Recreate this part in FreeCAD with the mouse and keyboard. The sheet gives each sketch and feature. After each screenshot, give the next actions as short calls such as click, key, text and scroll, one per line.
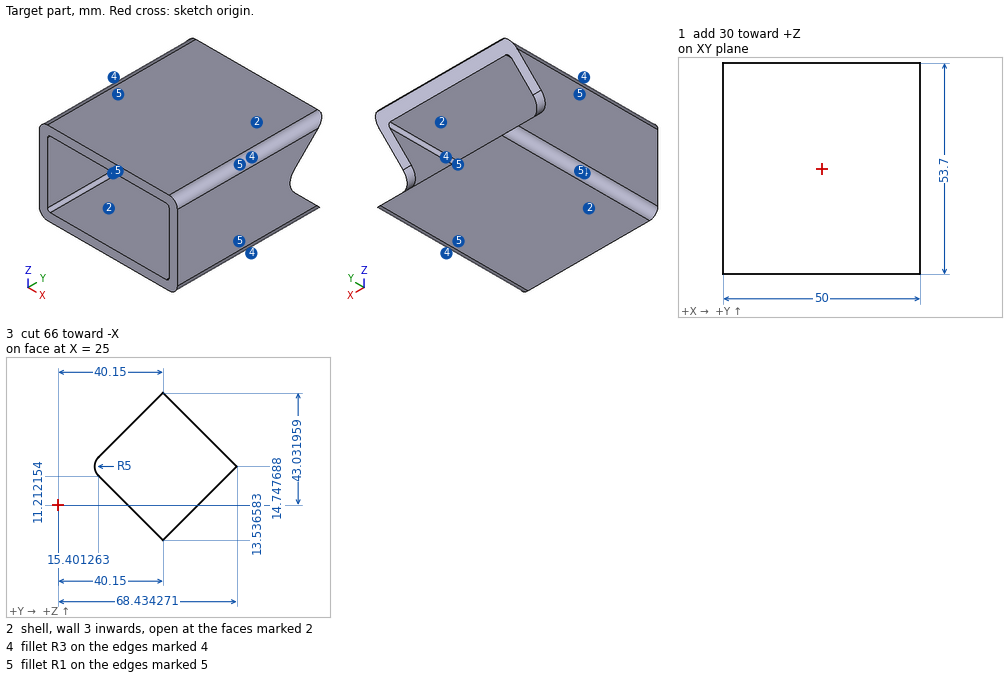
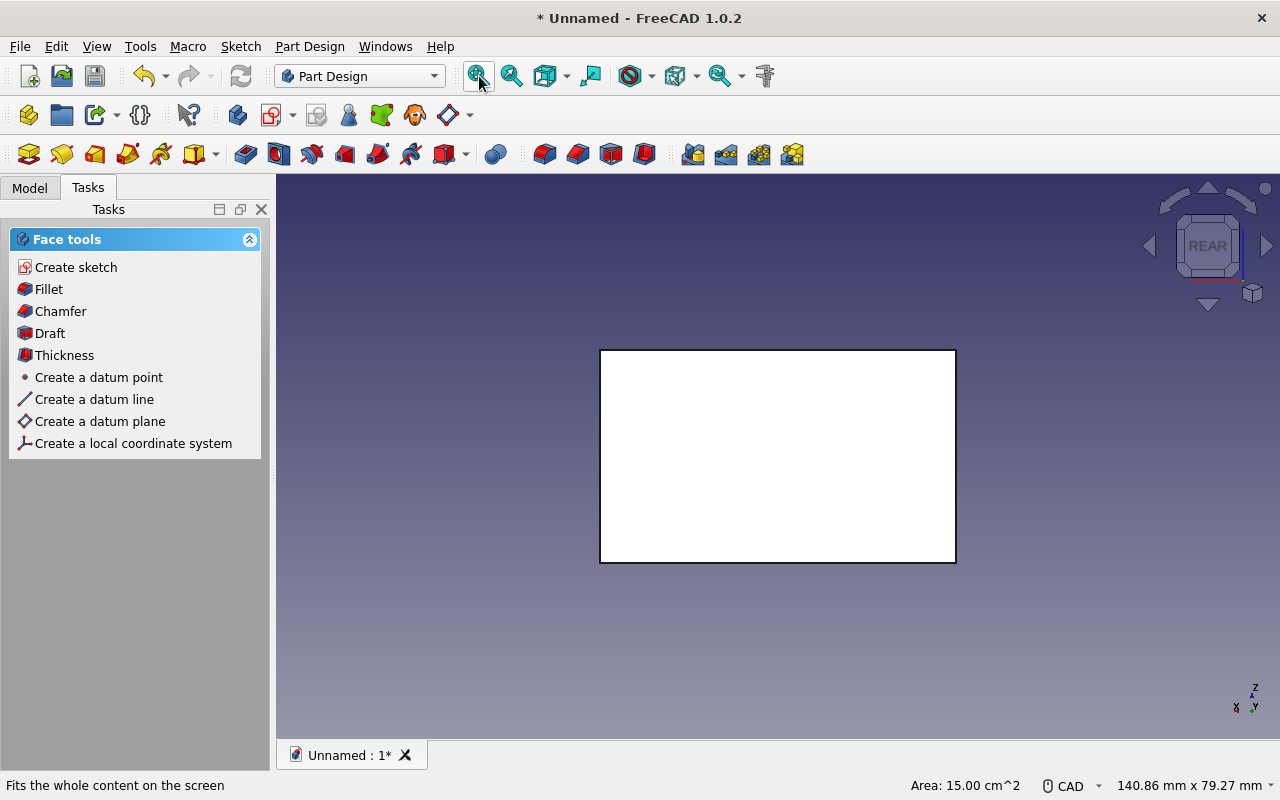
click(479, 76)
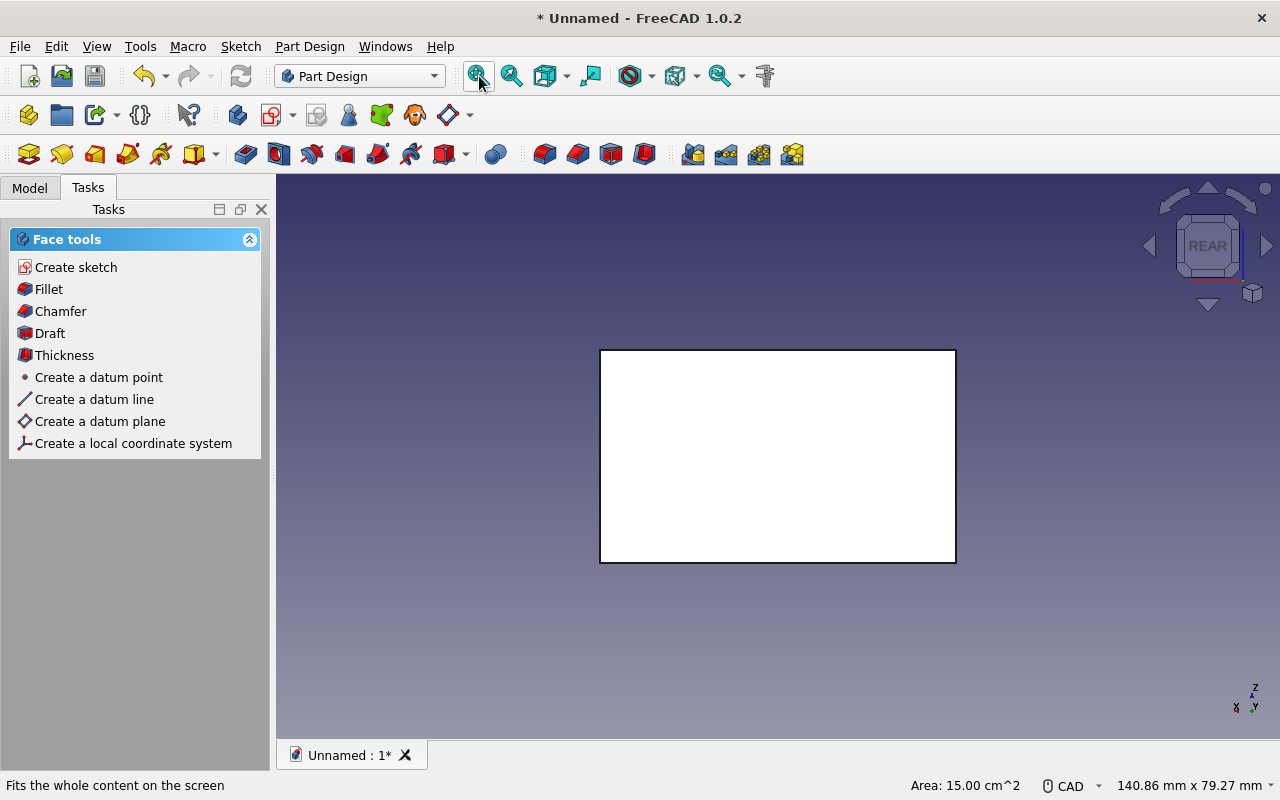
click(727, 456, ctrl)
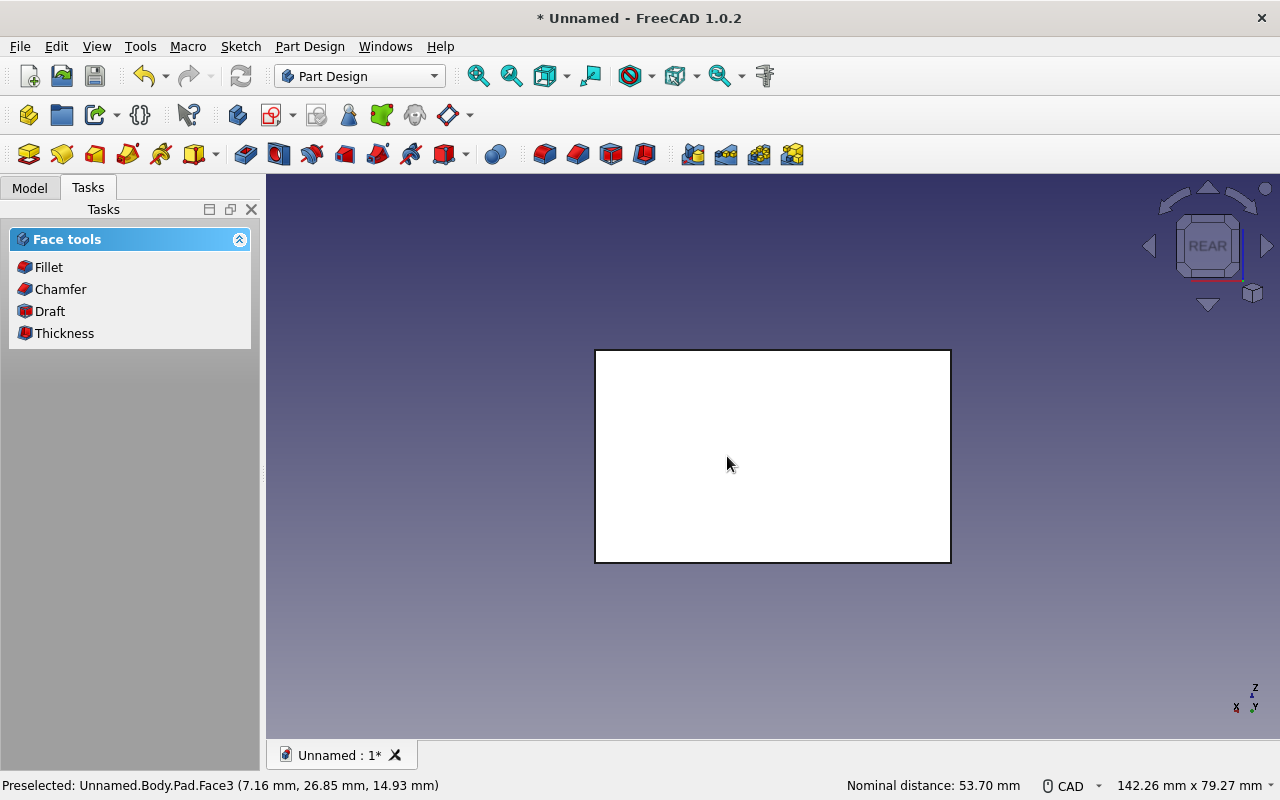
click(644, 154)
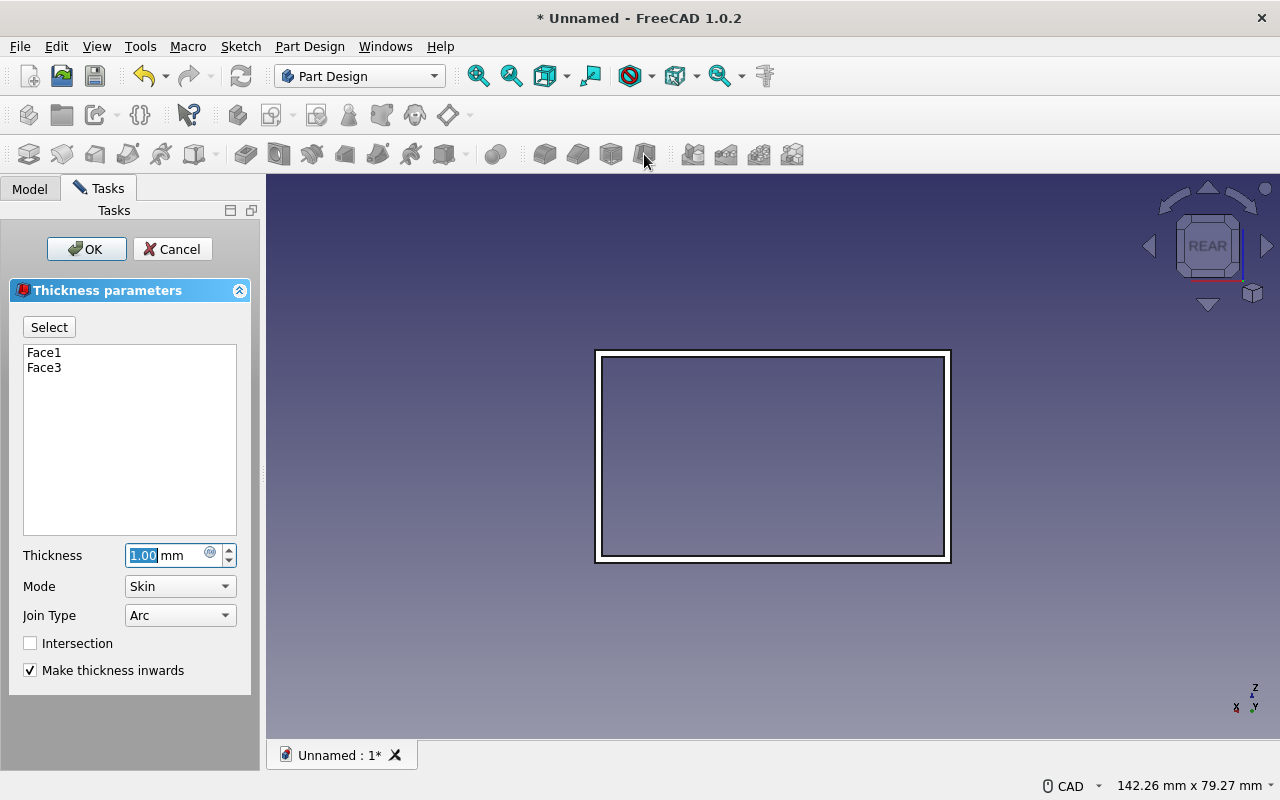
text(3)
key(Tab)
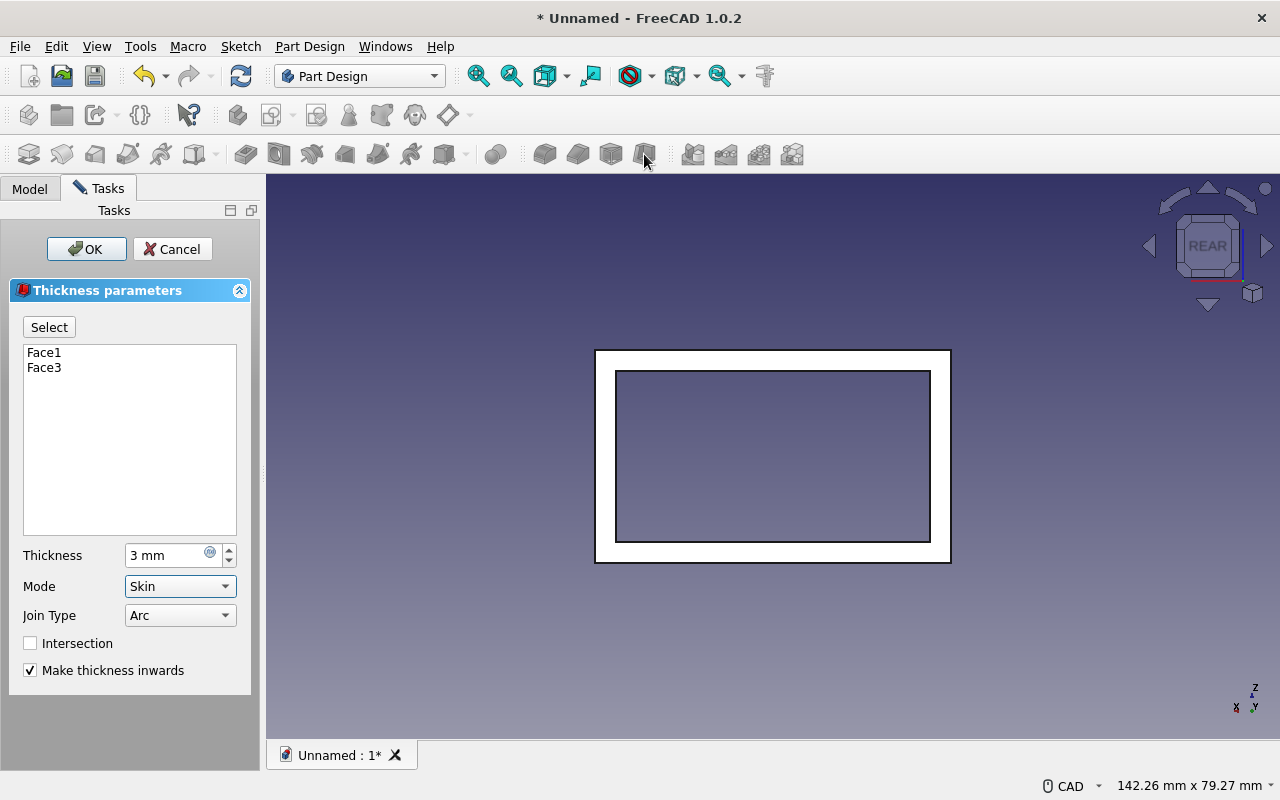
click(181, 616)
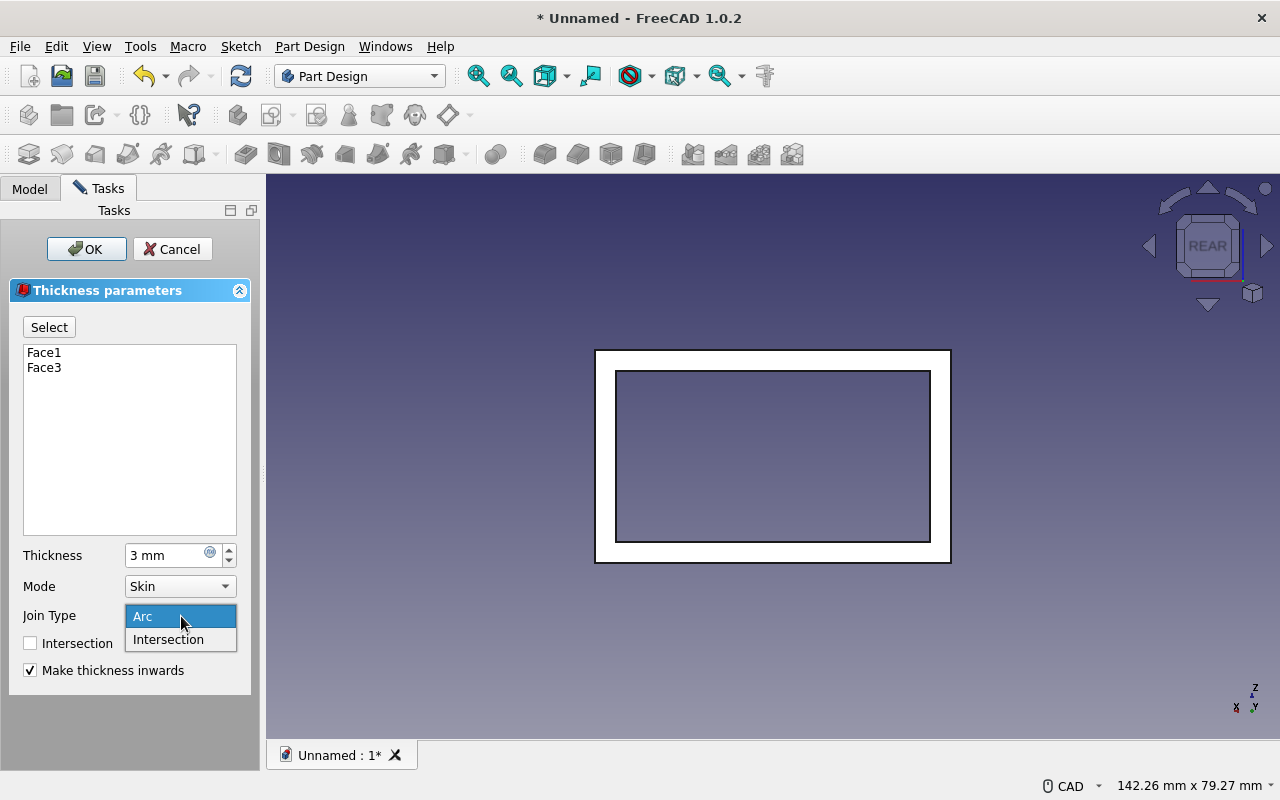
click(179, 640)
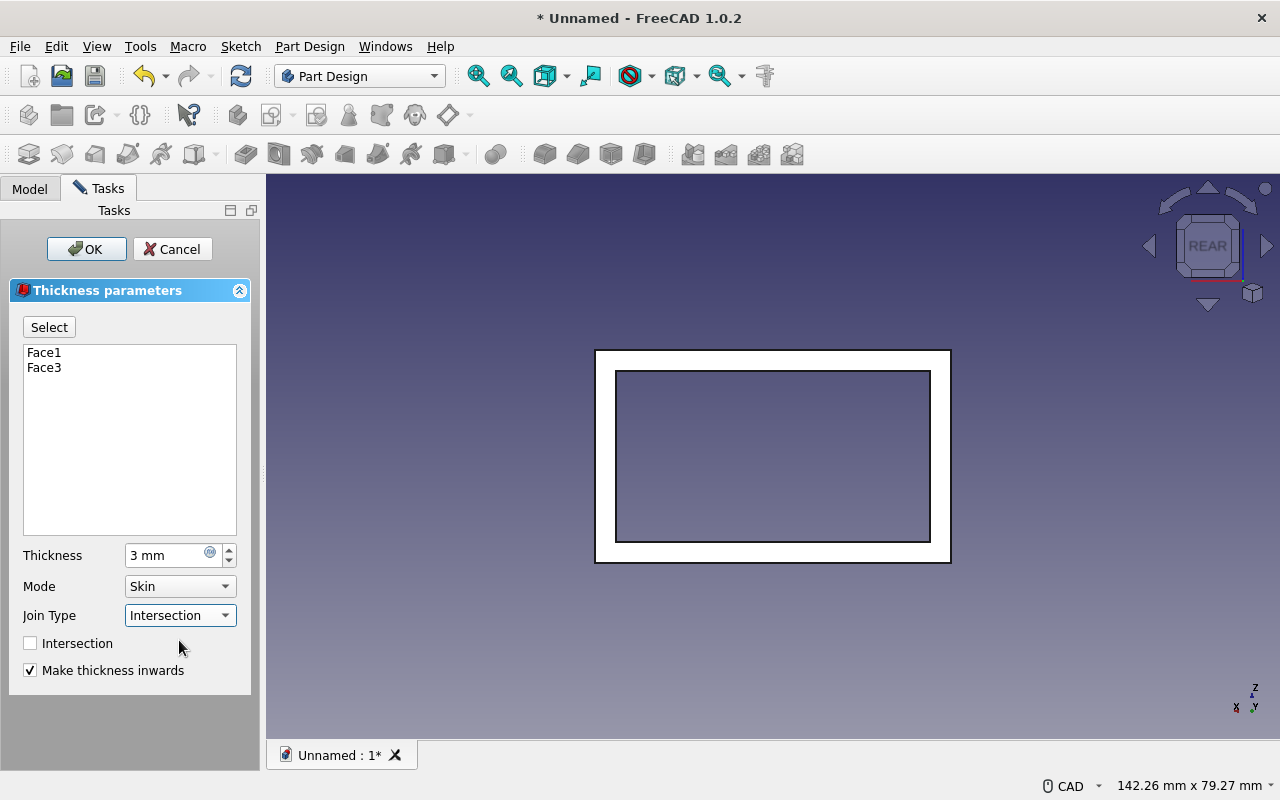
click(87, 249)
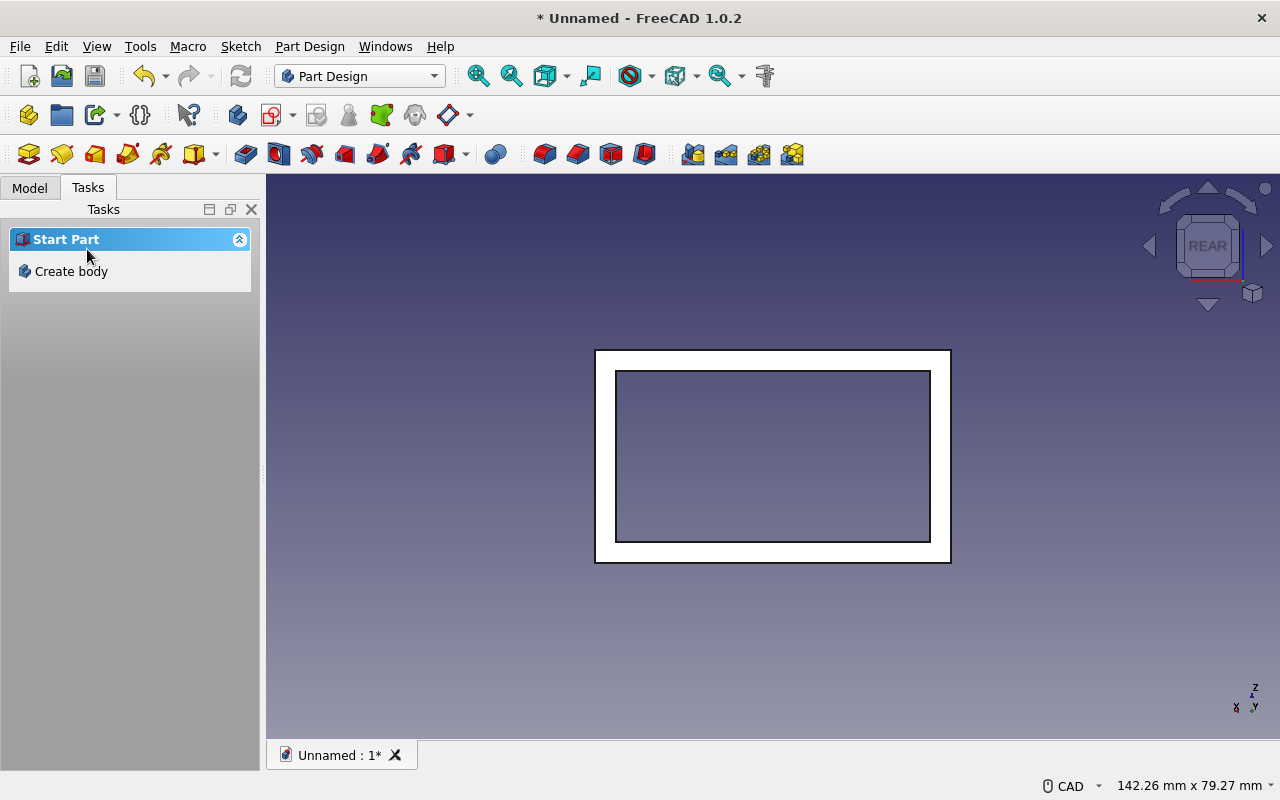
key(v)
key(f)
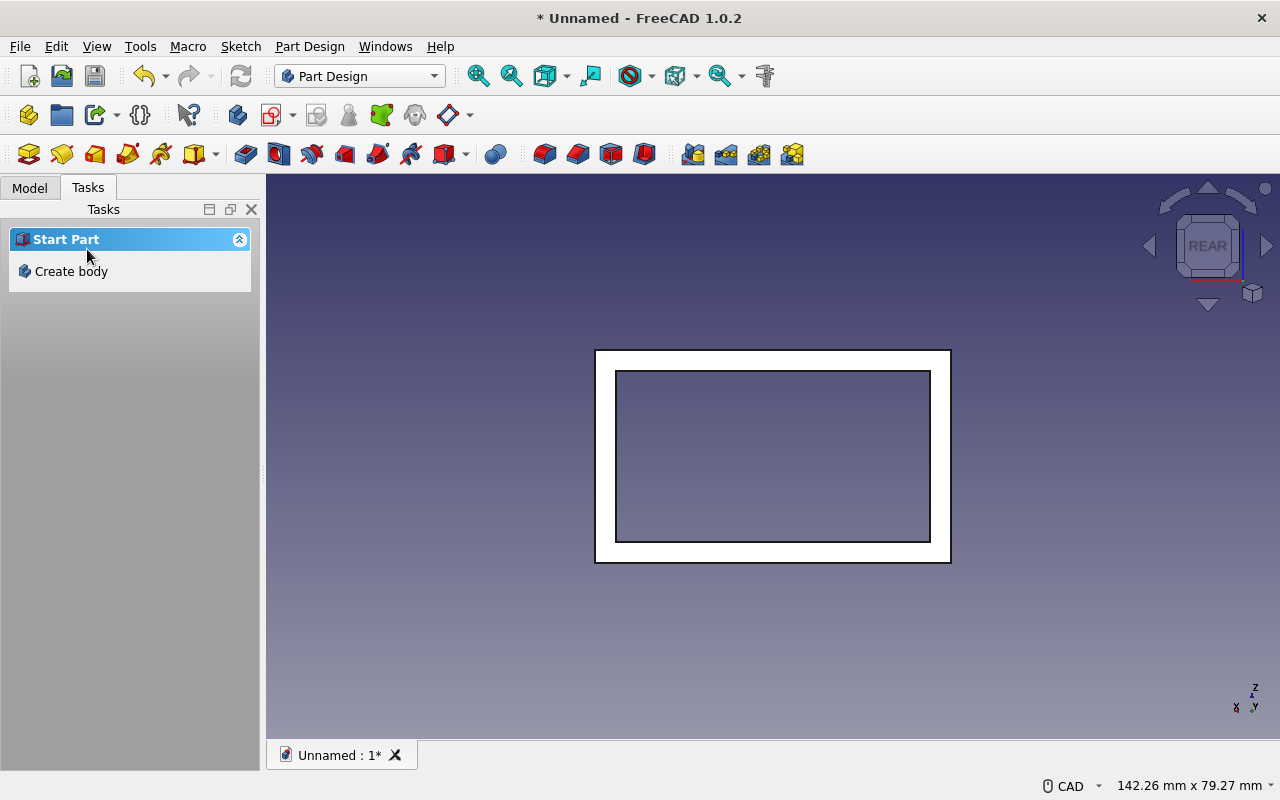
key(0)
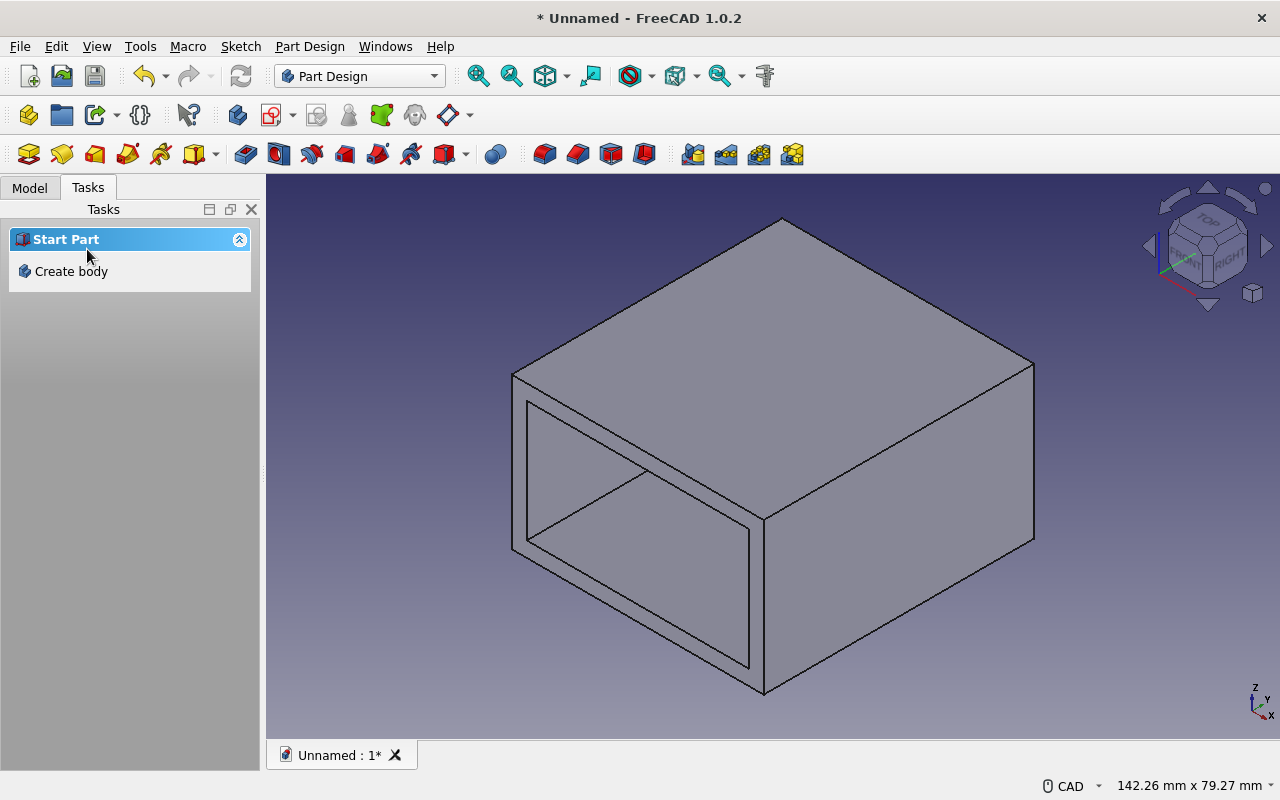
click(938, 506)